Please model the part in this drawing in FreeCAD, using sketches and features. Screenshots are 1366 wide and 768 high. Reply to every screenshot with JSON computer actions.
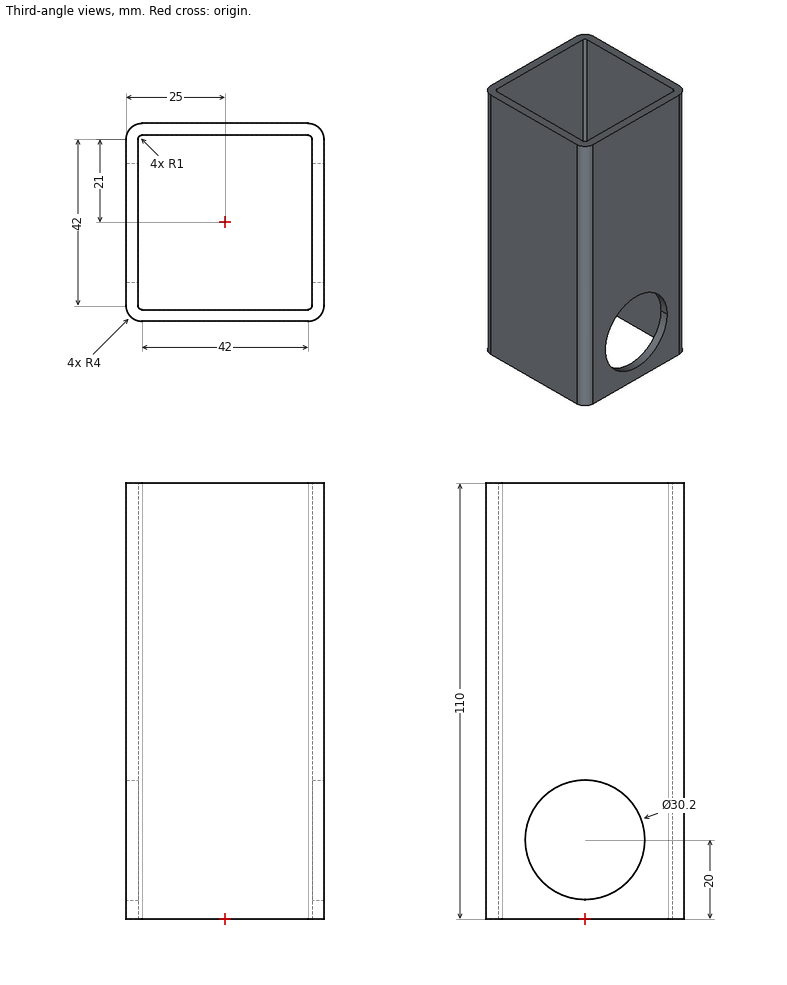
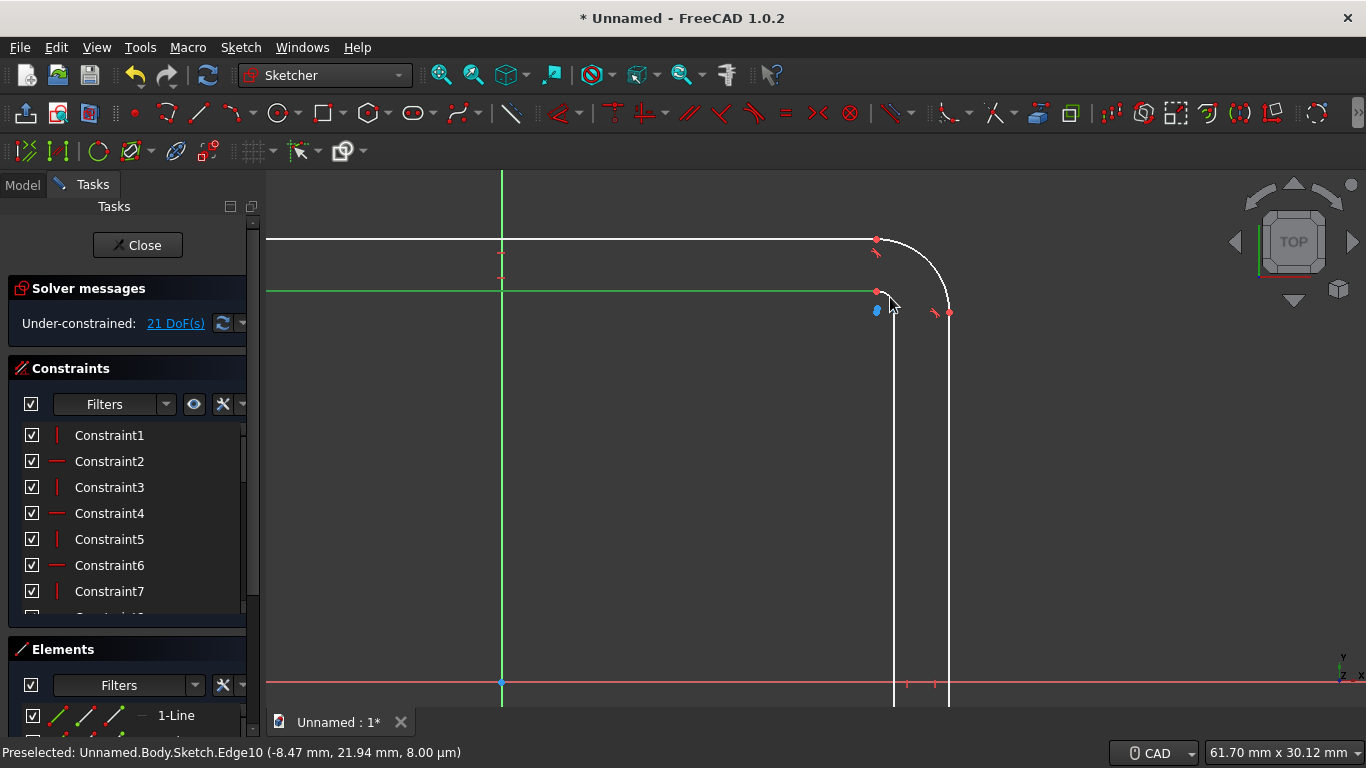
{"action": "left_click", "coordinate": [890, 296]}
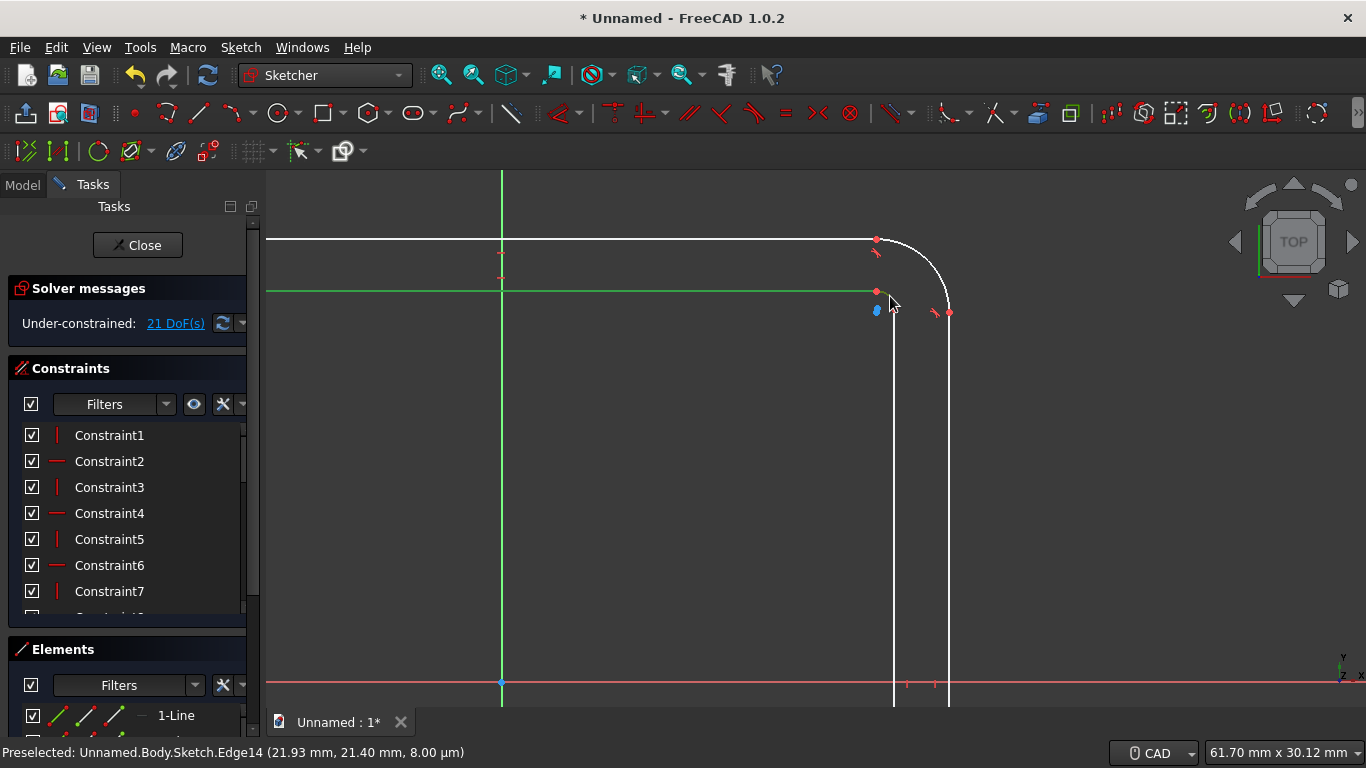
{"action": "left_click", "coordinate": [754, 114]}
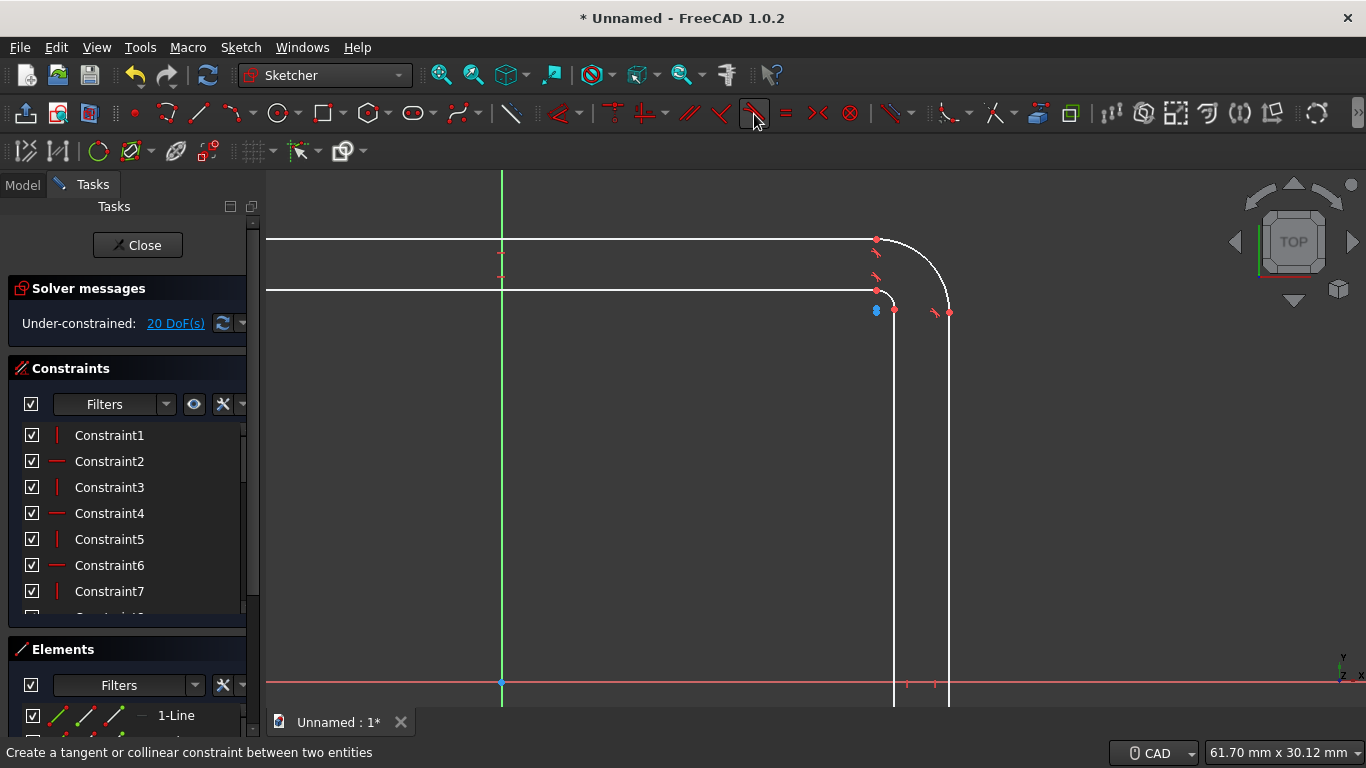
{"action": "left_click", "coordinate": [894, 534]}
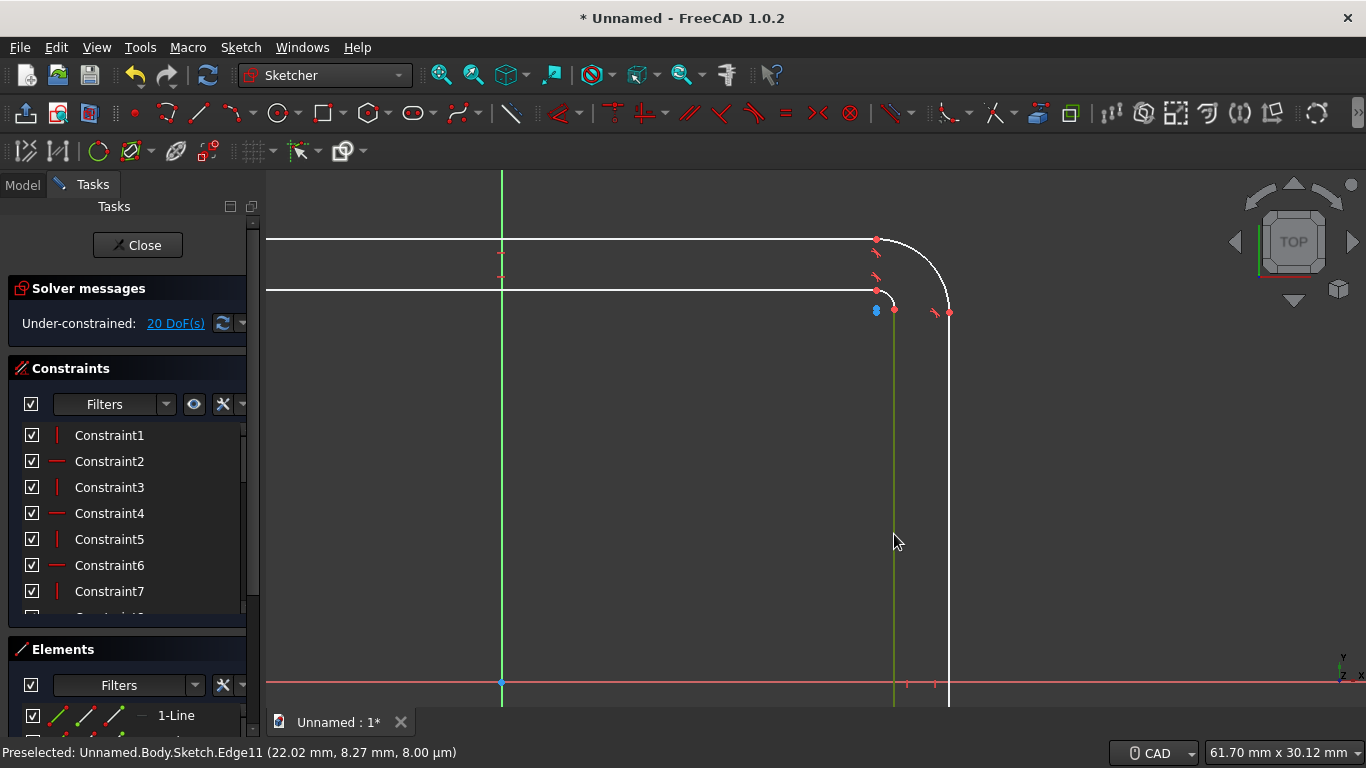
{"action": "left_click", "coordinate": [890, 296]}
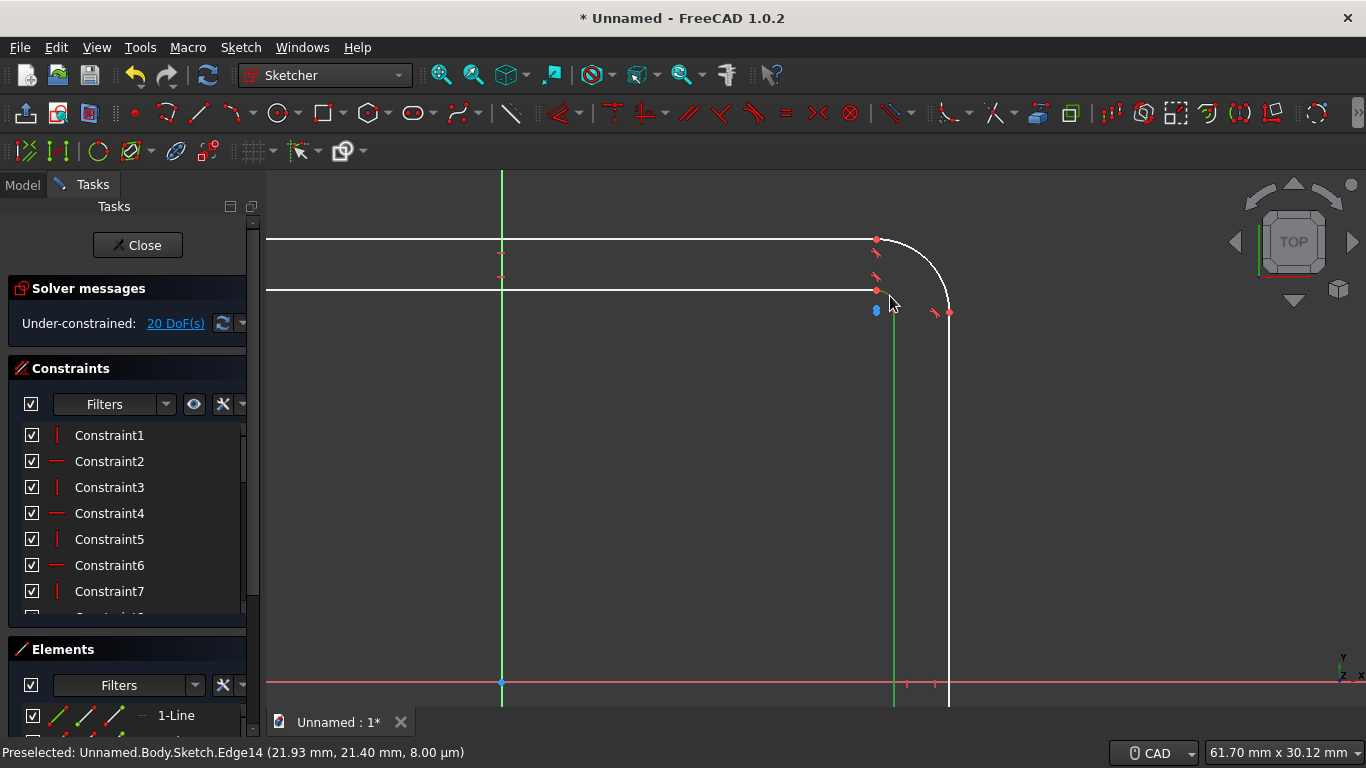
{"action": "left_click", "coordinate": [754, 114]}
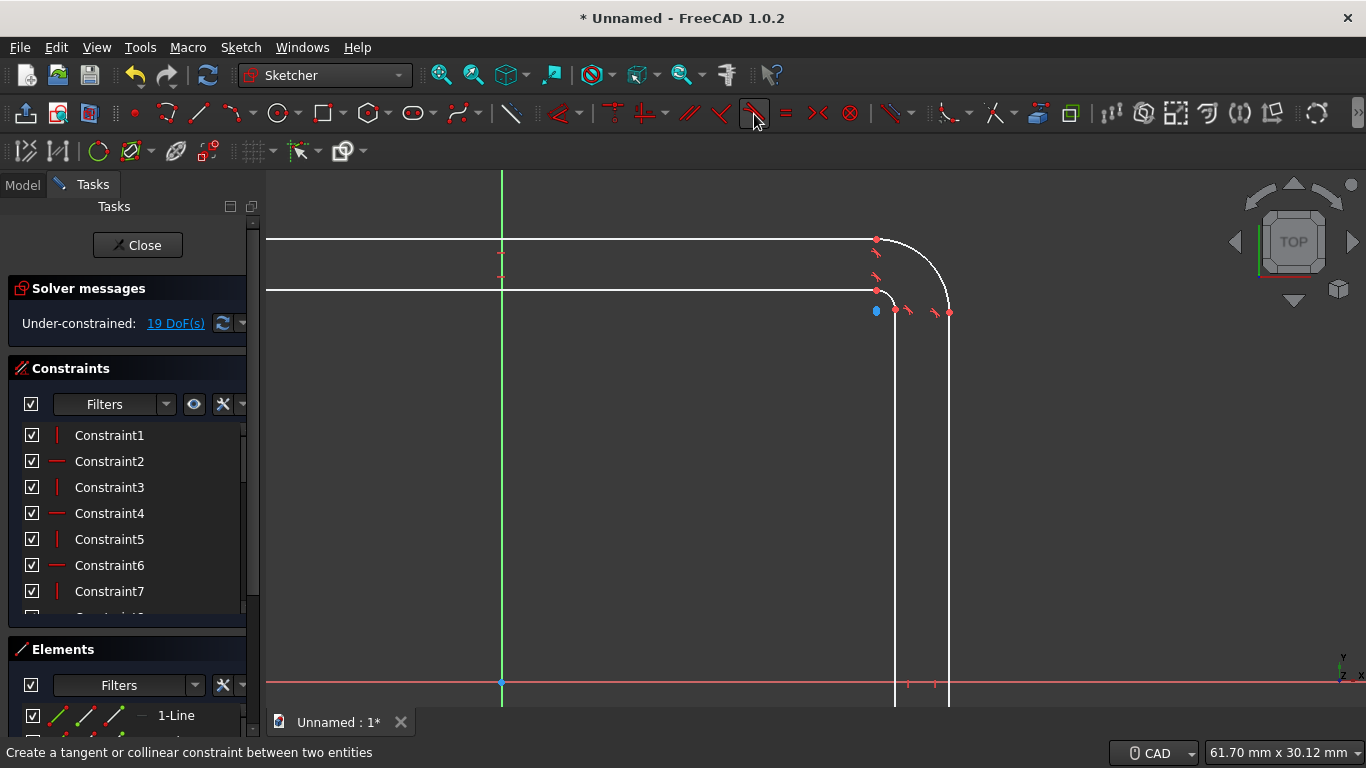
{"action": "left_click", "coordinate": [895, 534]}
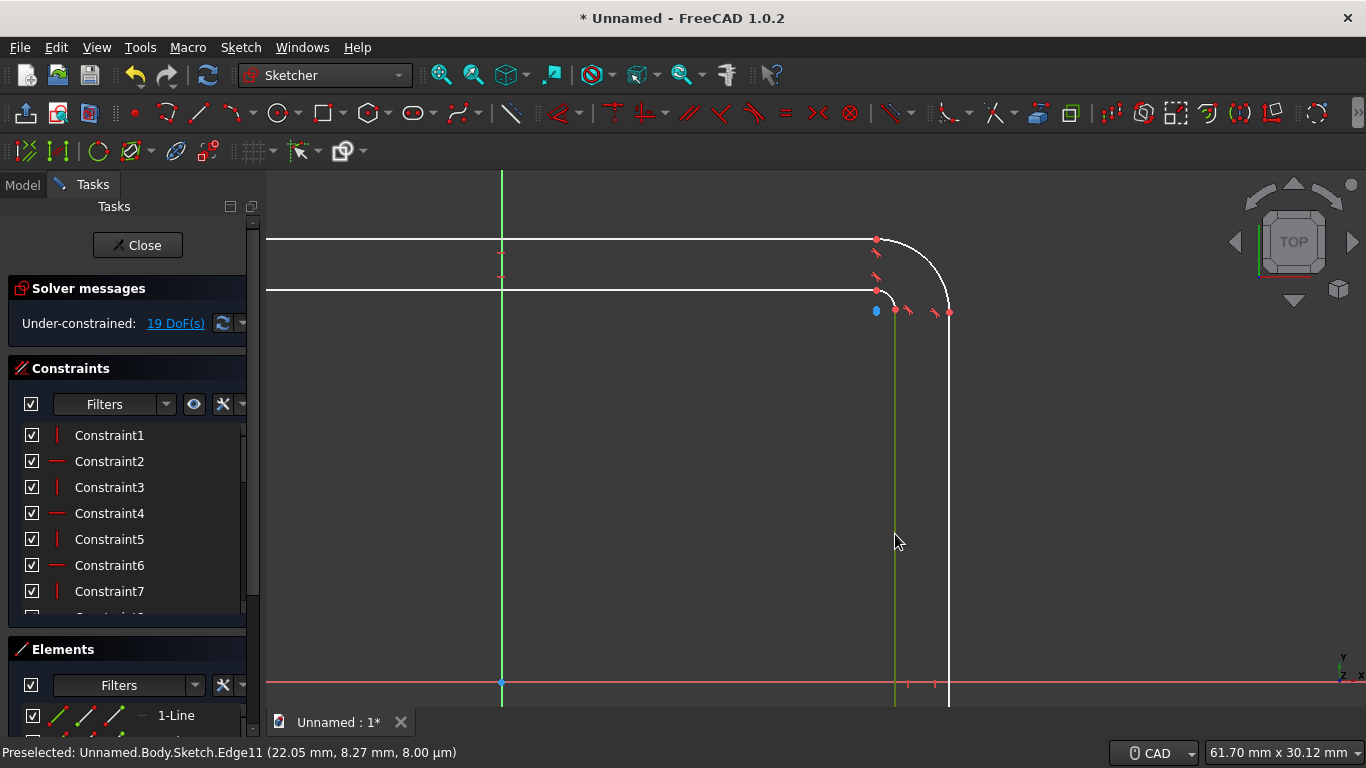
{"action": "scroll", "coordinate": [890, 297], "scroll_direction": "down", "scroll_amount": 5}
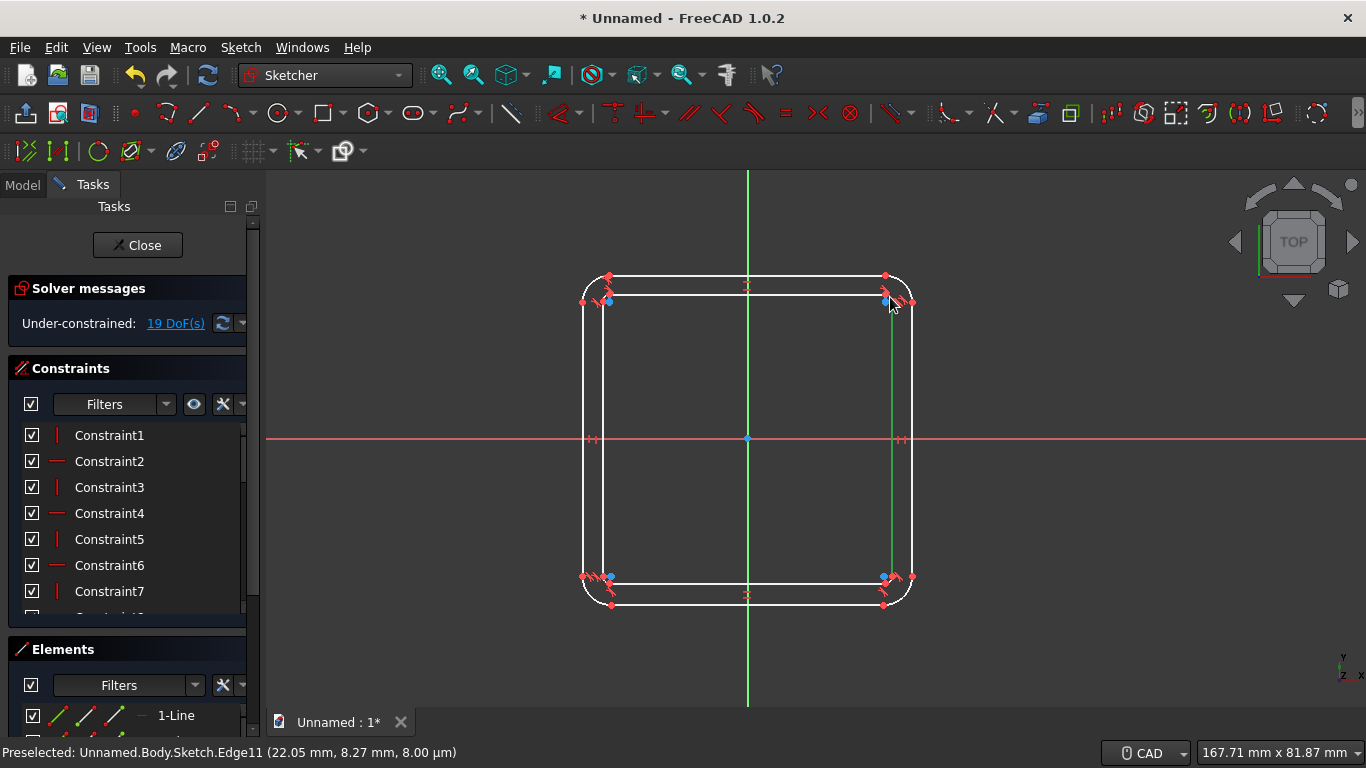
{"action": "scroll", "coordinate": [890, 582], "scroll_direction": "up", "scroll_amount": 5}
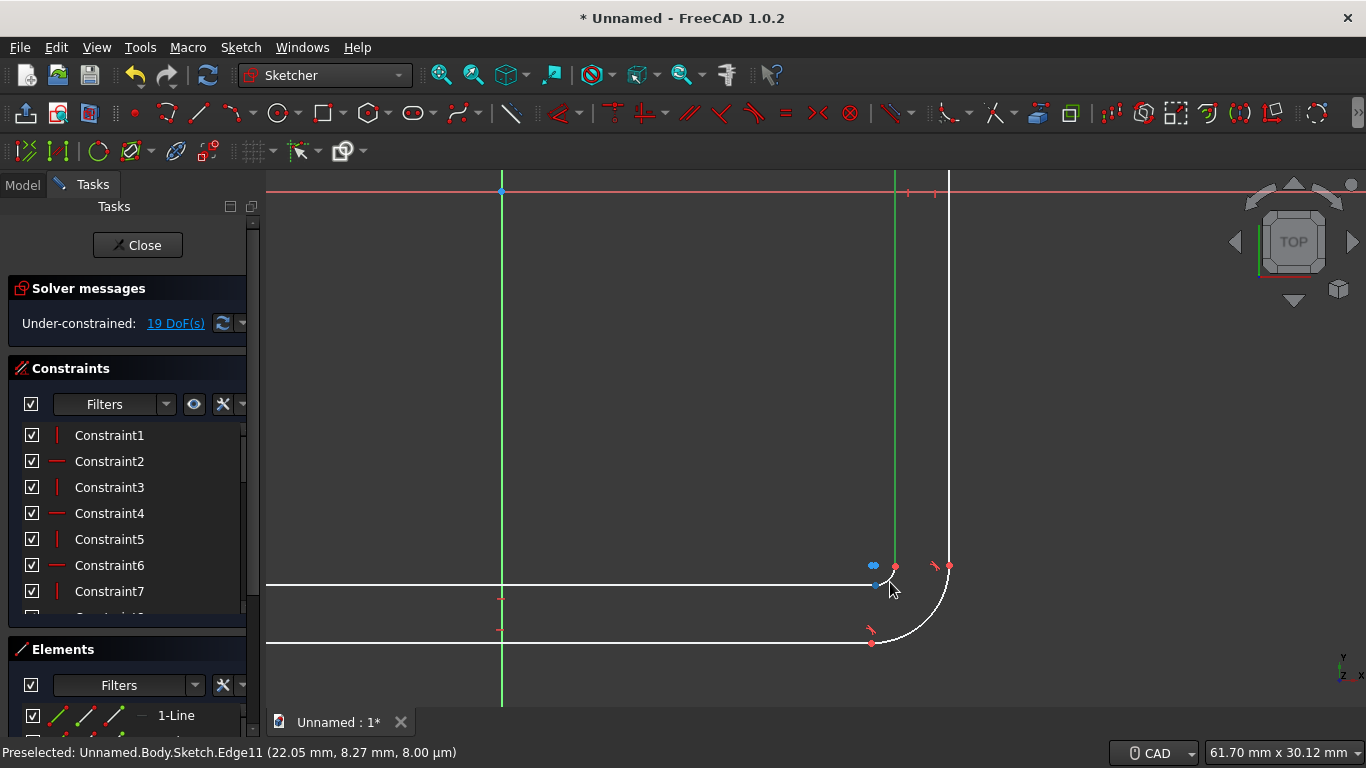
{"action": "left_click", "coordinate": [889, 580]}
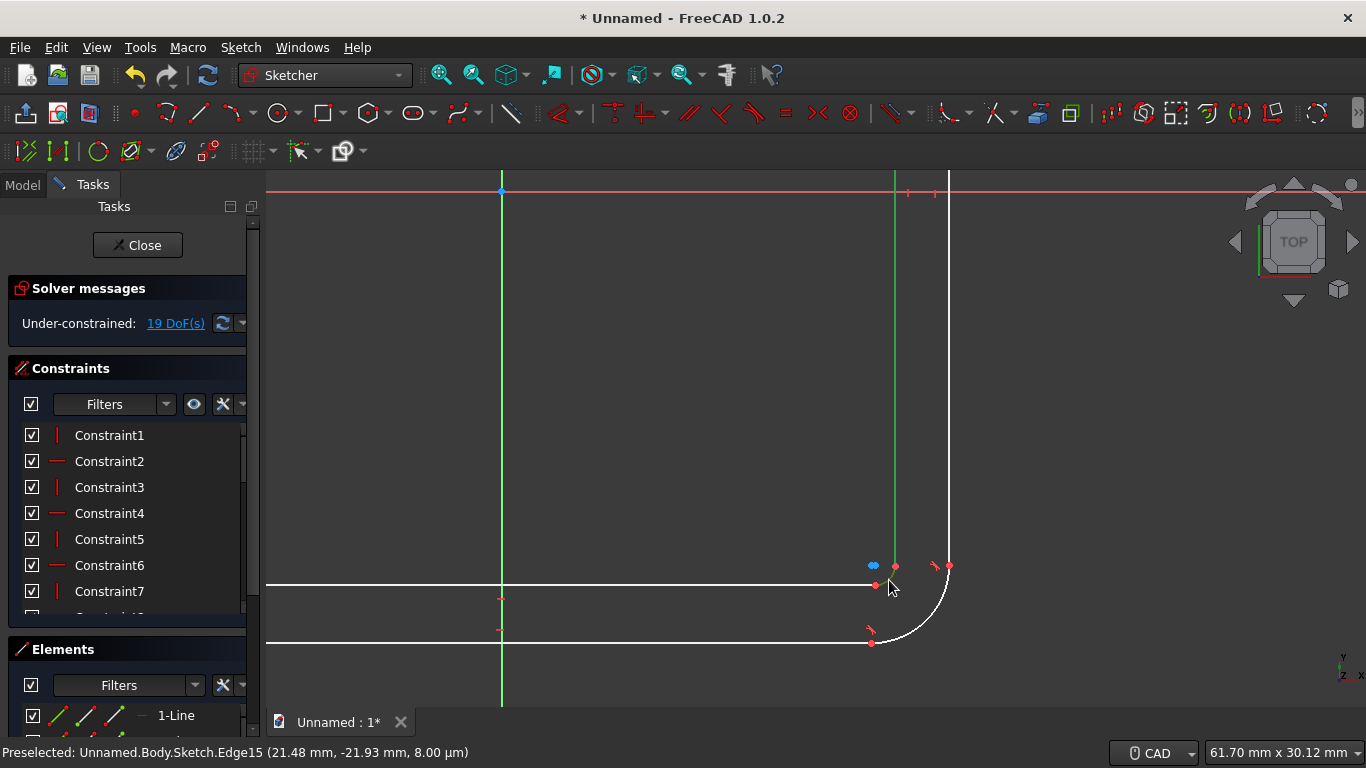
{"action": "left_click", "coordinate": [754, 114]}